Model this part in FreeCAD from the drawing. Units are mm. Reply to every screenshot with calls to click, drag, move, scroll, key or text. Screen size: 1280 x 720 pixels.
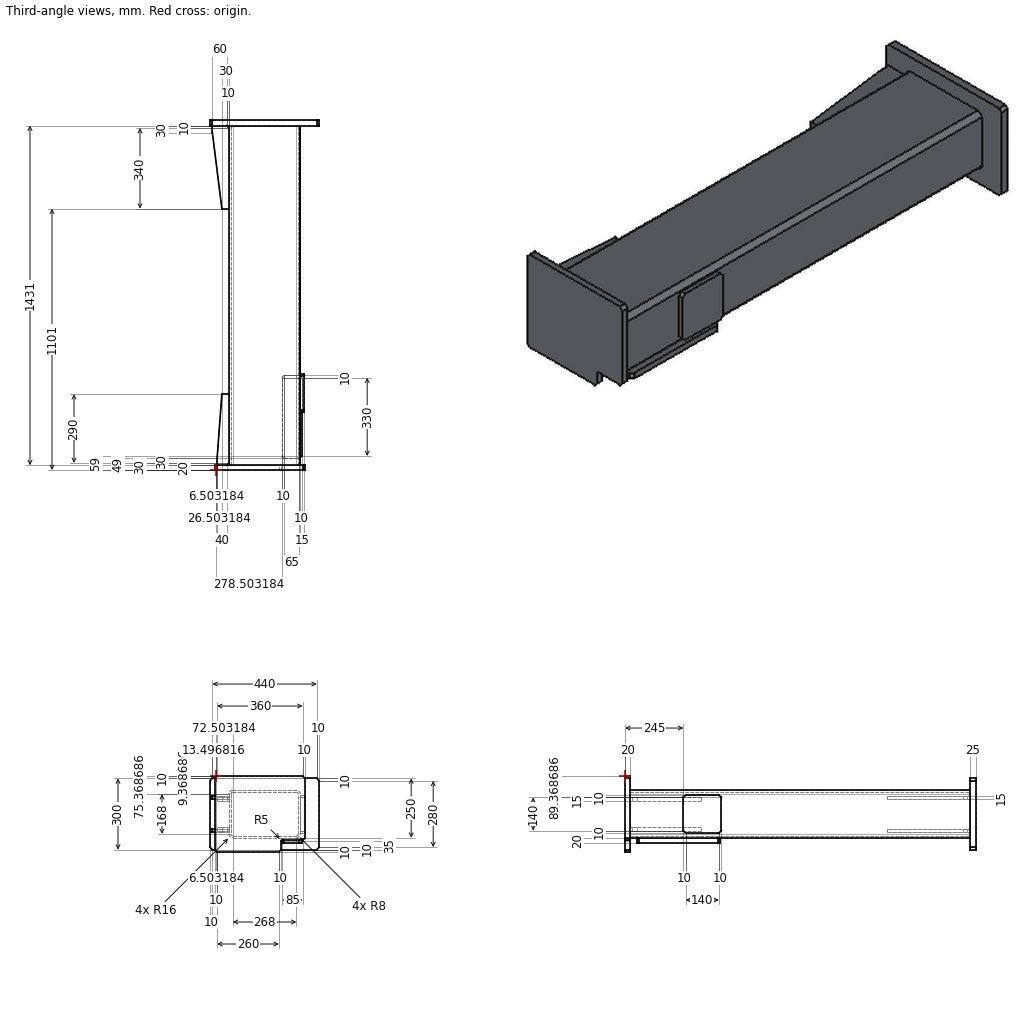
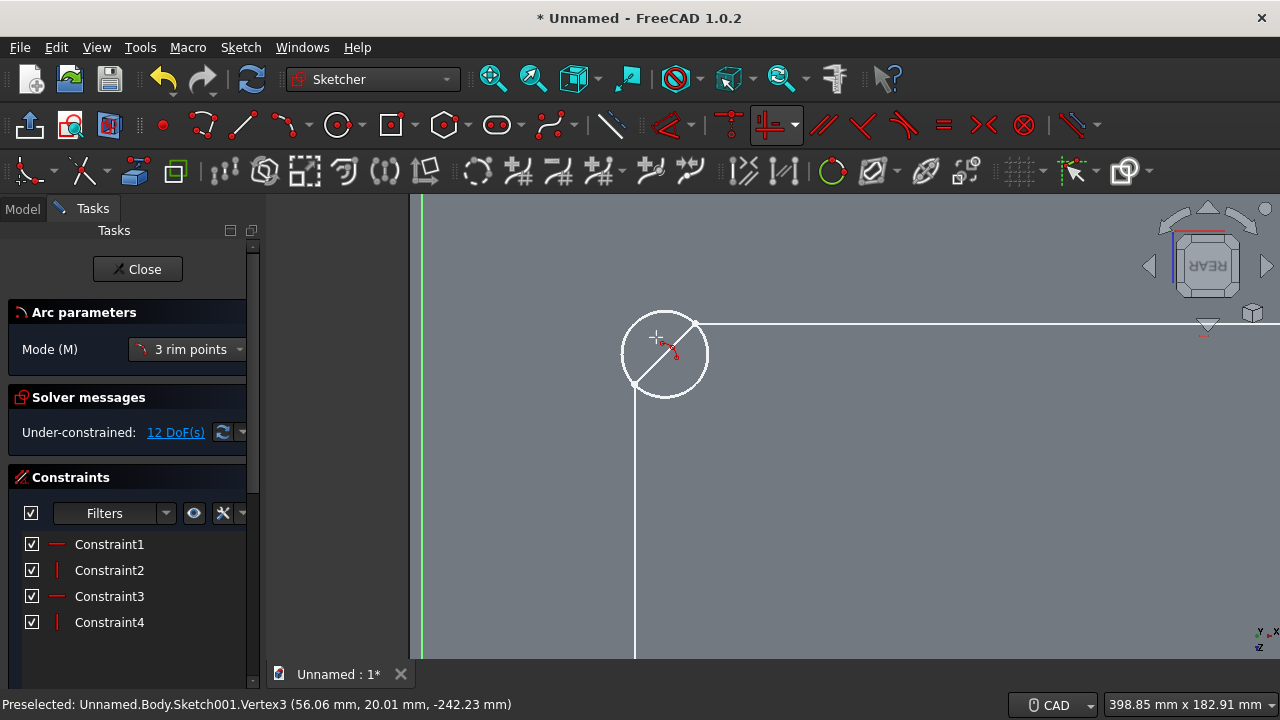
click(654, 338)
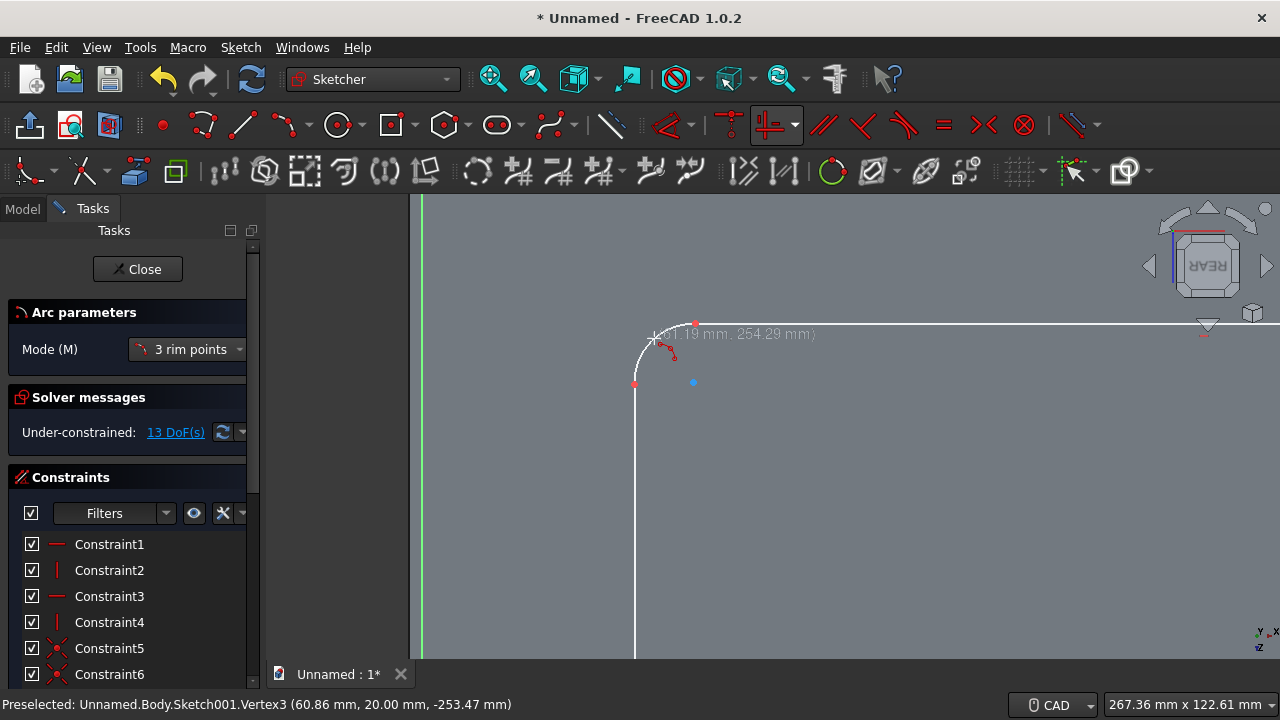
scroll(535, 261, down, 6)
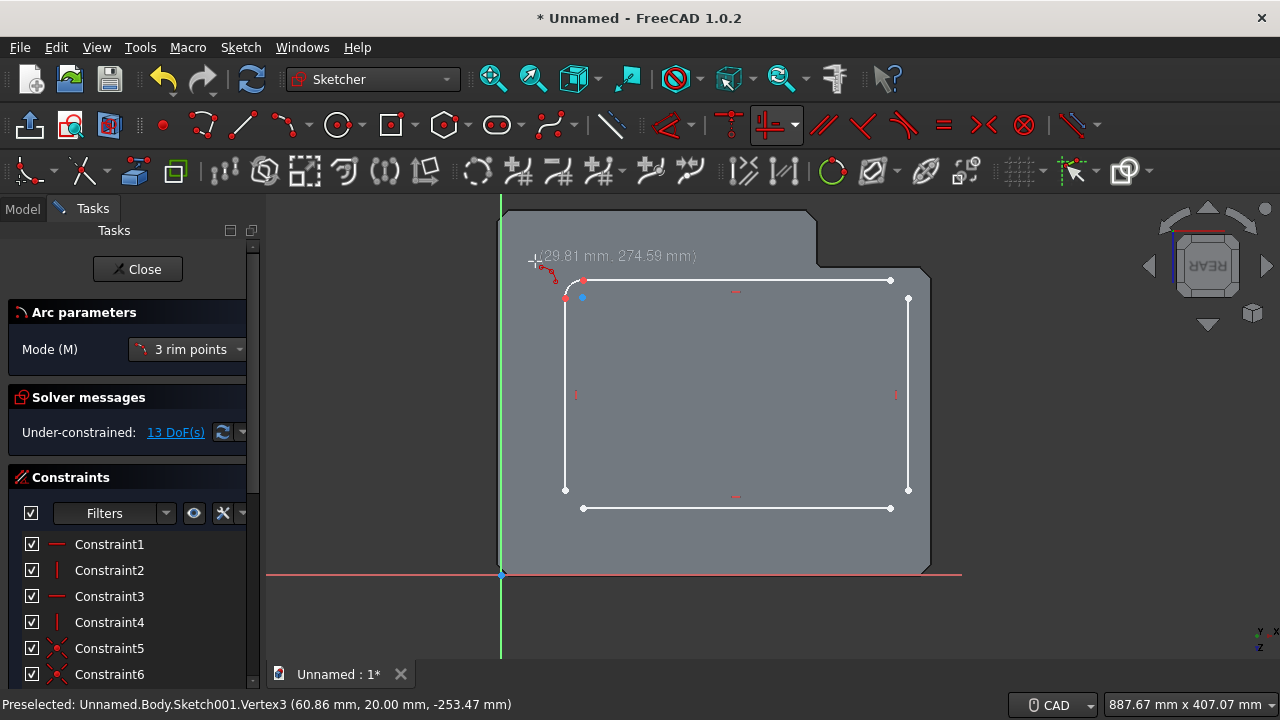
click(565, 490)
click(583, 508)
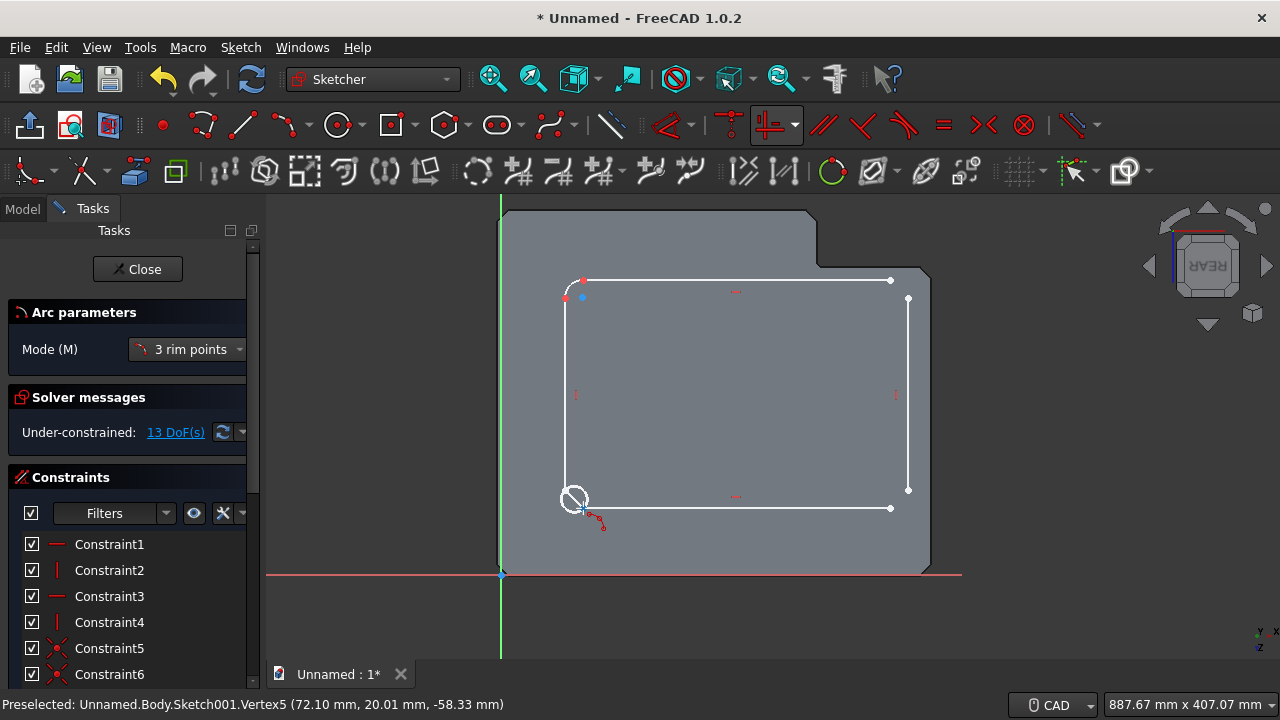
scroll(571, 502, up, 6)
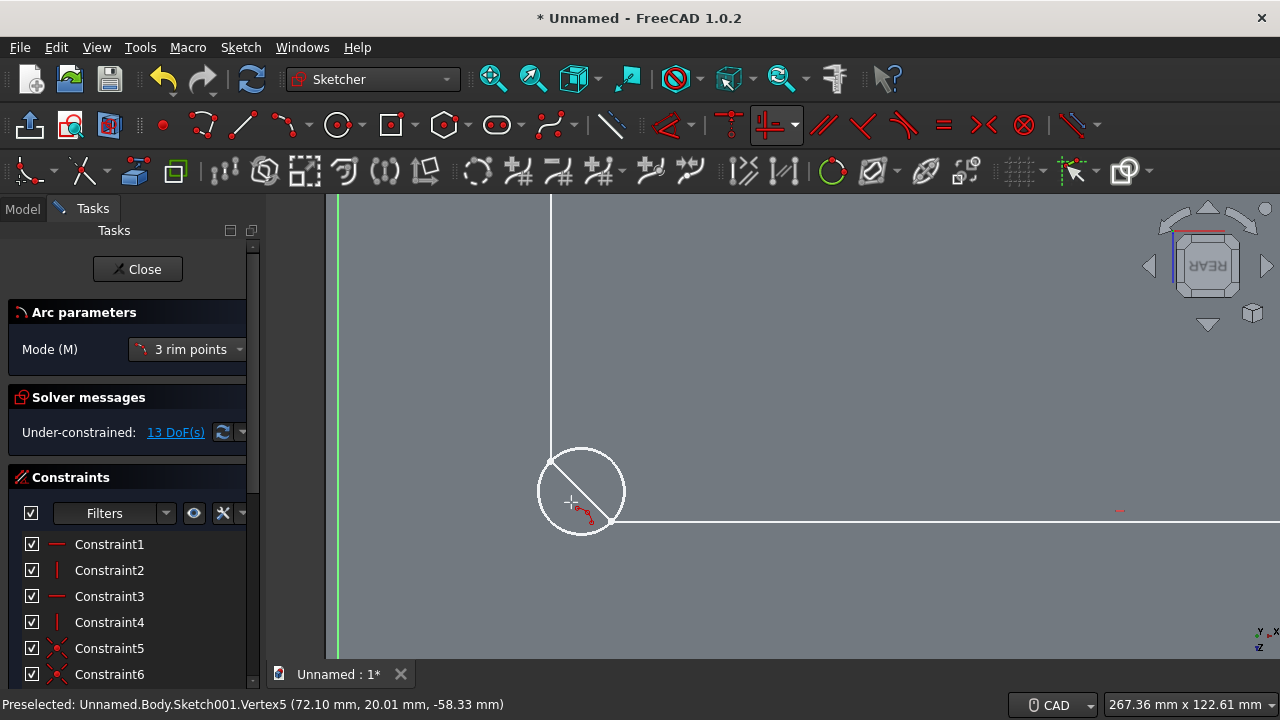
click(570, 500)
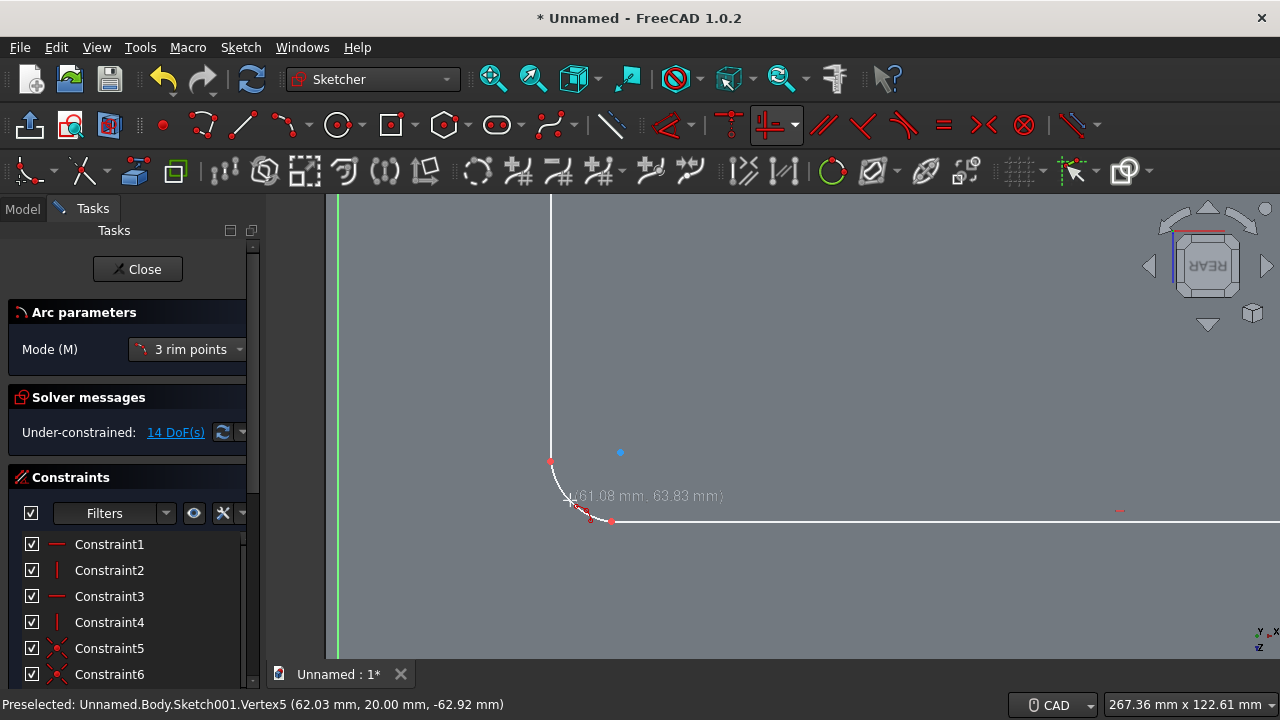
scroll(571, 502, down, 6)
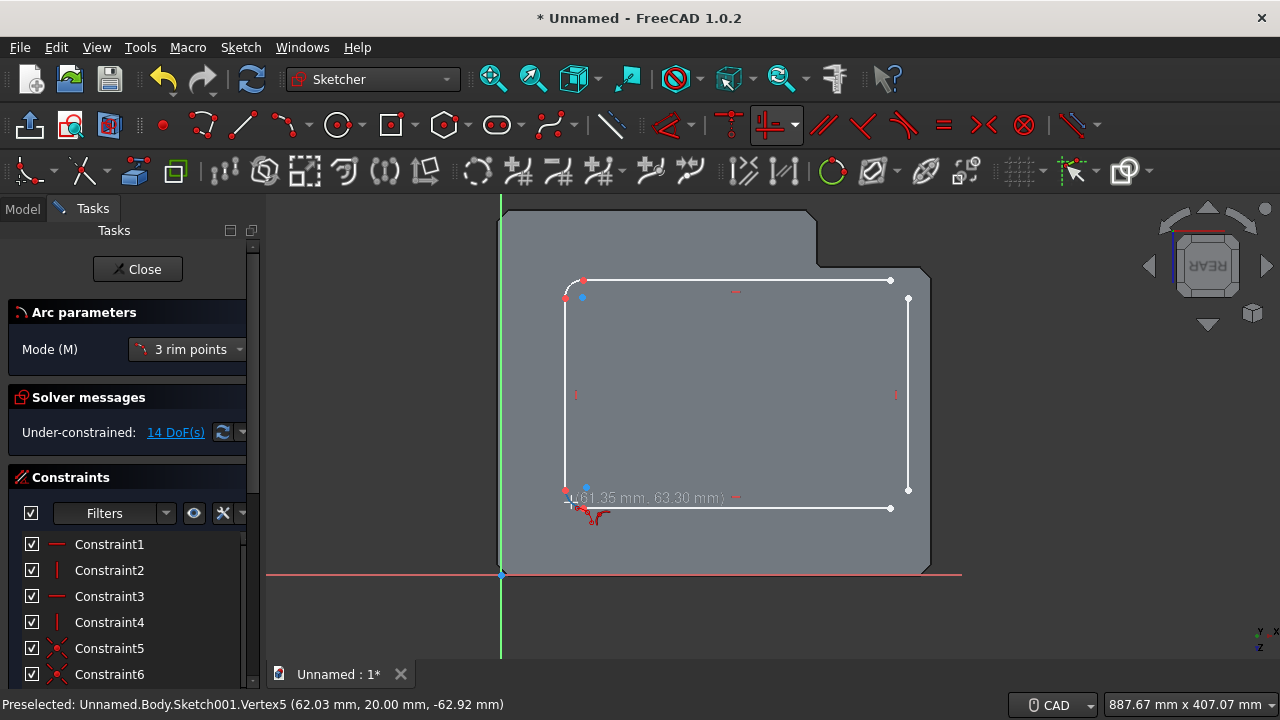
click(890, 508)
click(908, 490)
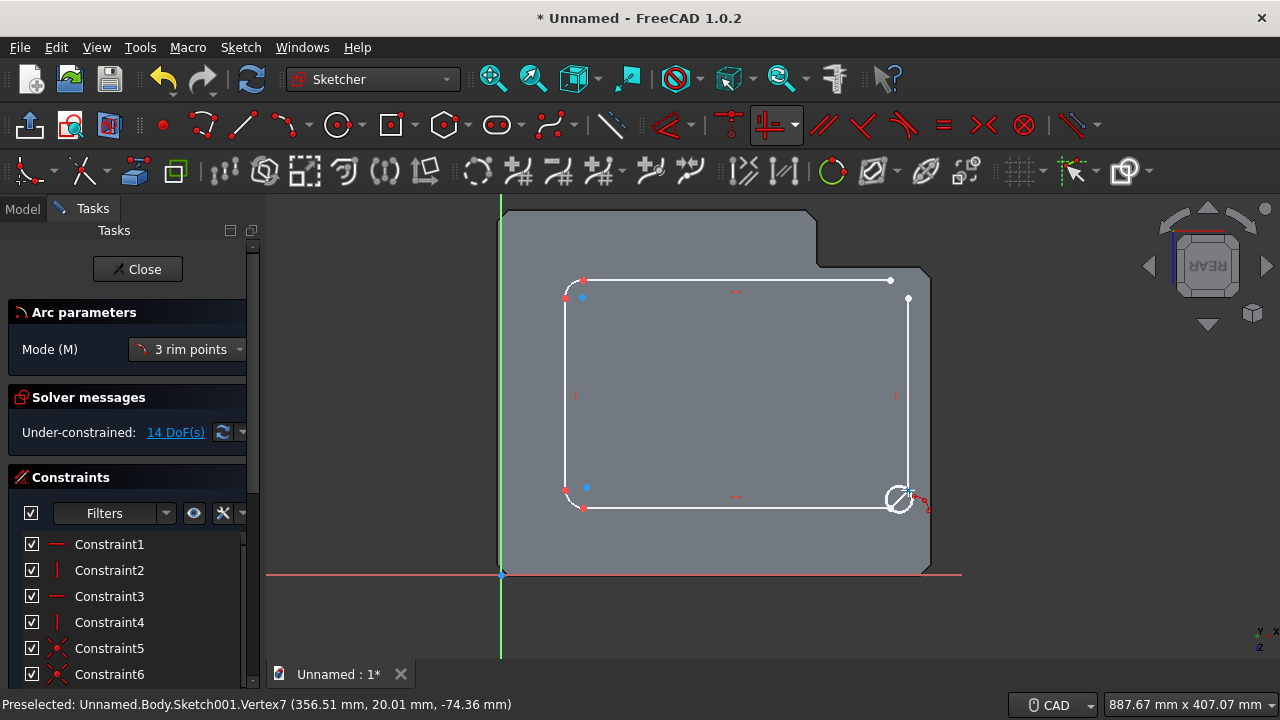
scroll(903, 502, up, 6)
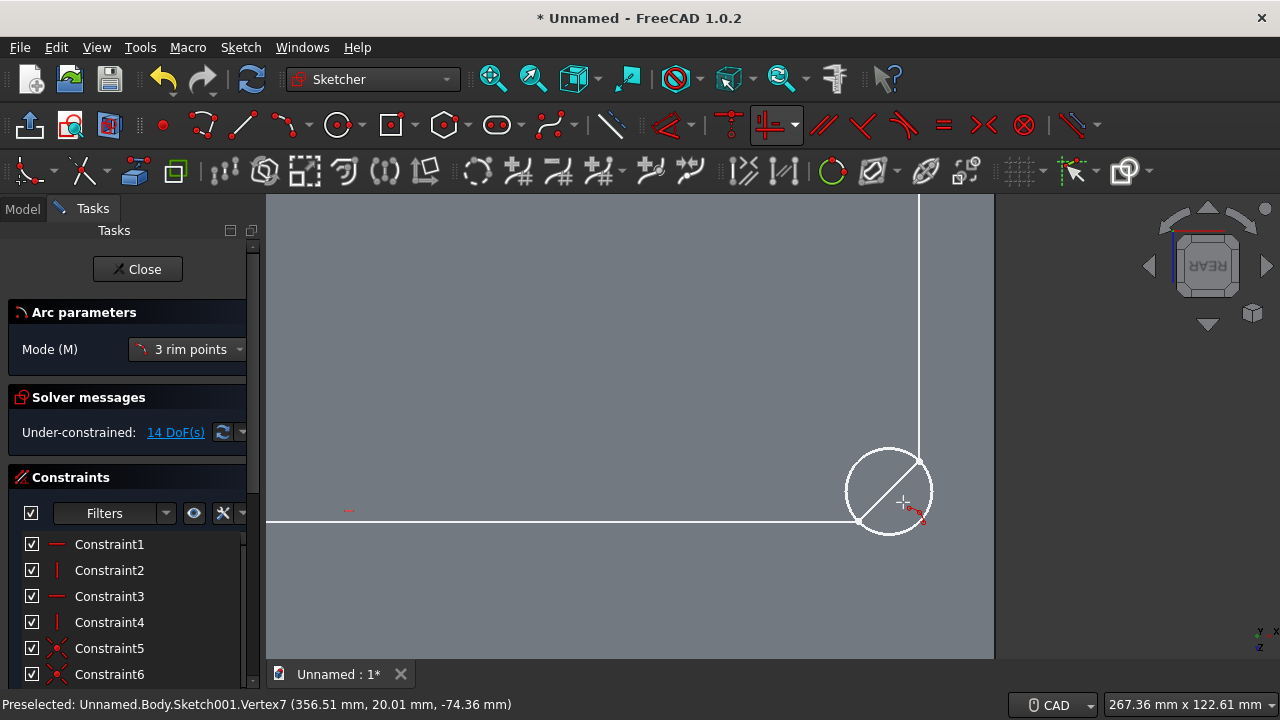
click(902, 500)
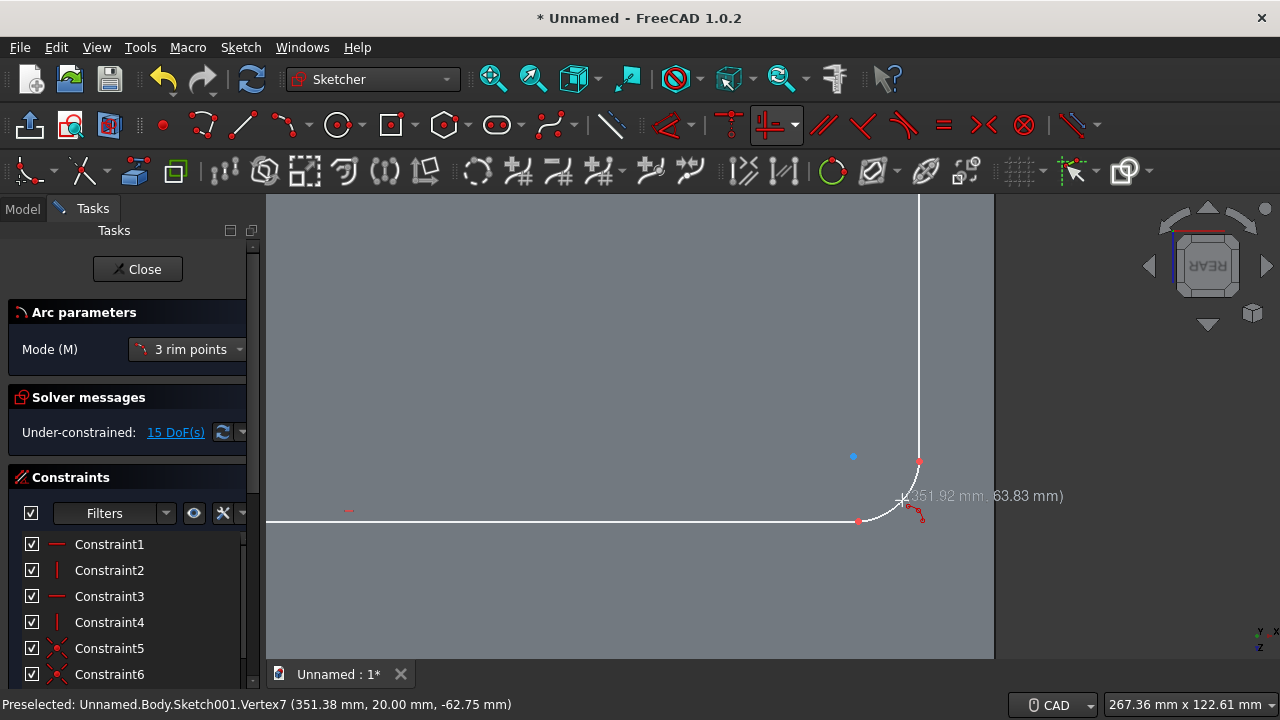
scroll(903, 502, down, 6)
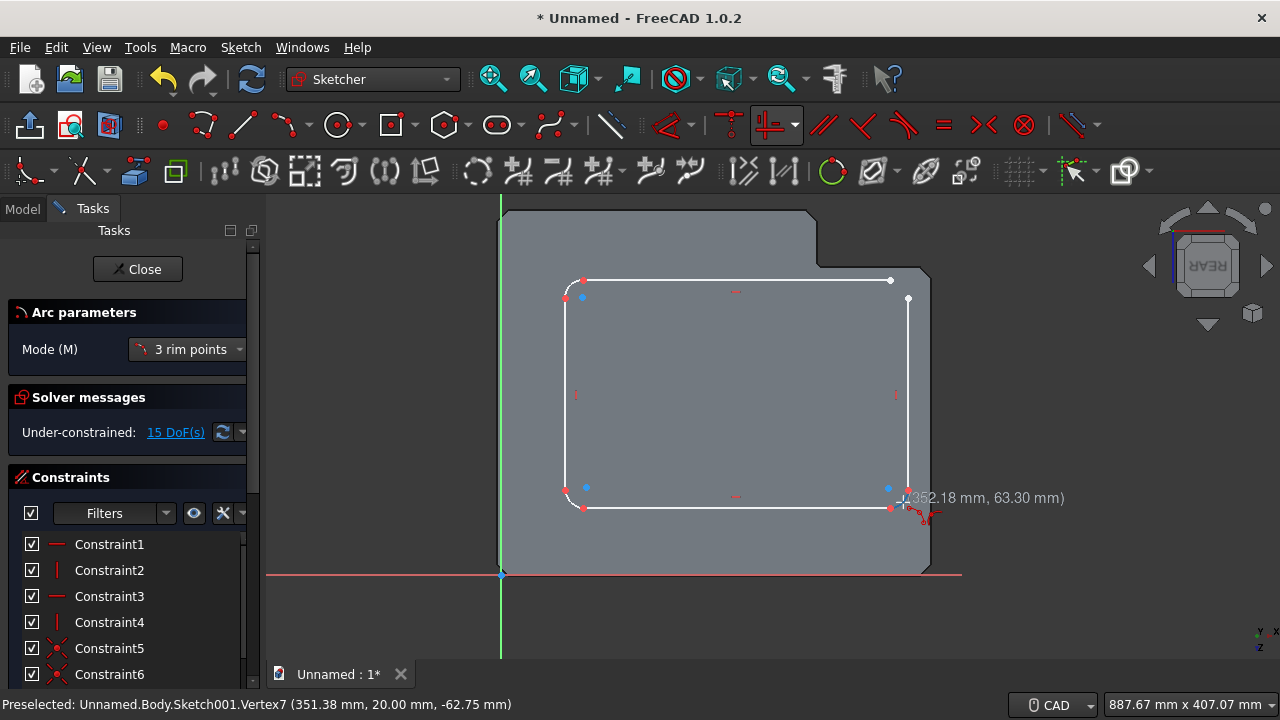
click(908, 298)
click(890, 280)